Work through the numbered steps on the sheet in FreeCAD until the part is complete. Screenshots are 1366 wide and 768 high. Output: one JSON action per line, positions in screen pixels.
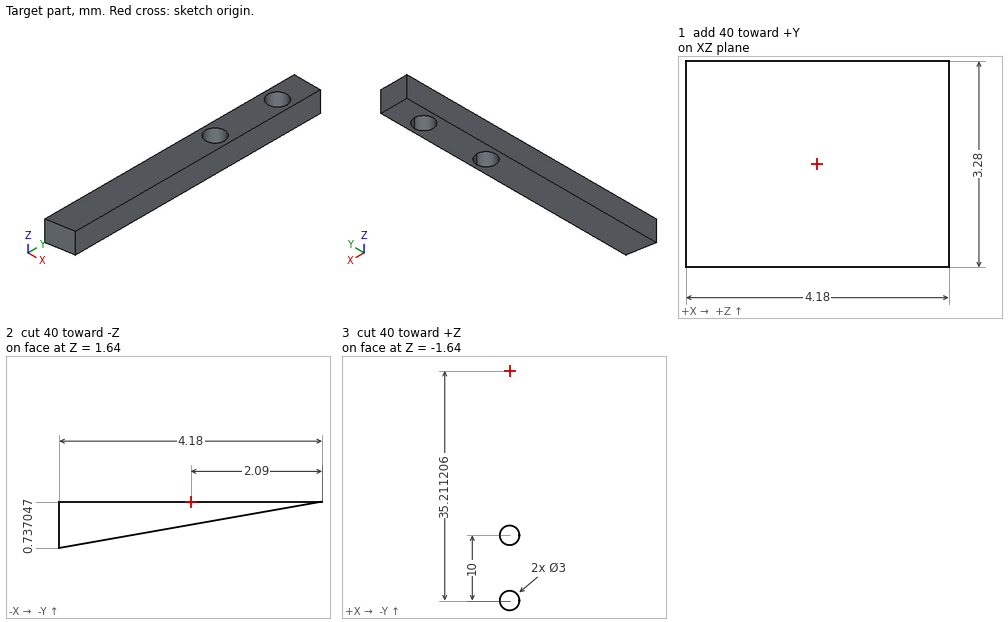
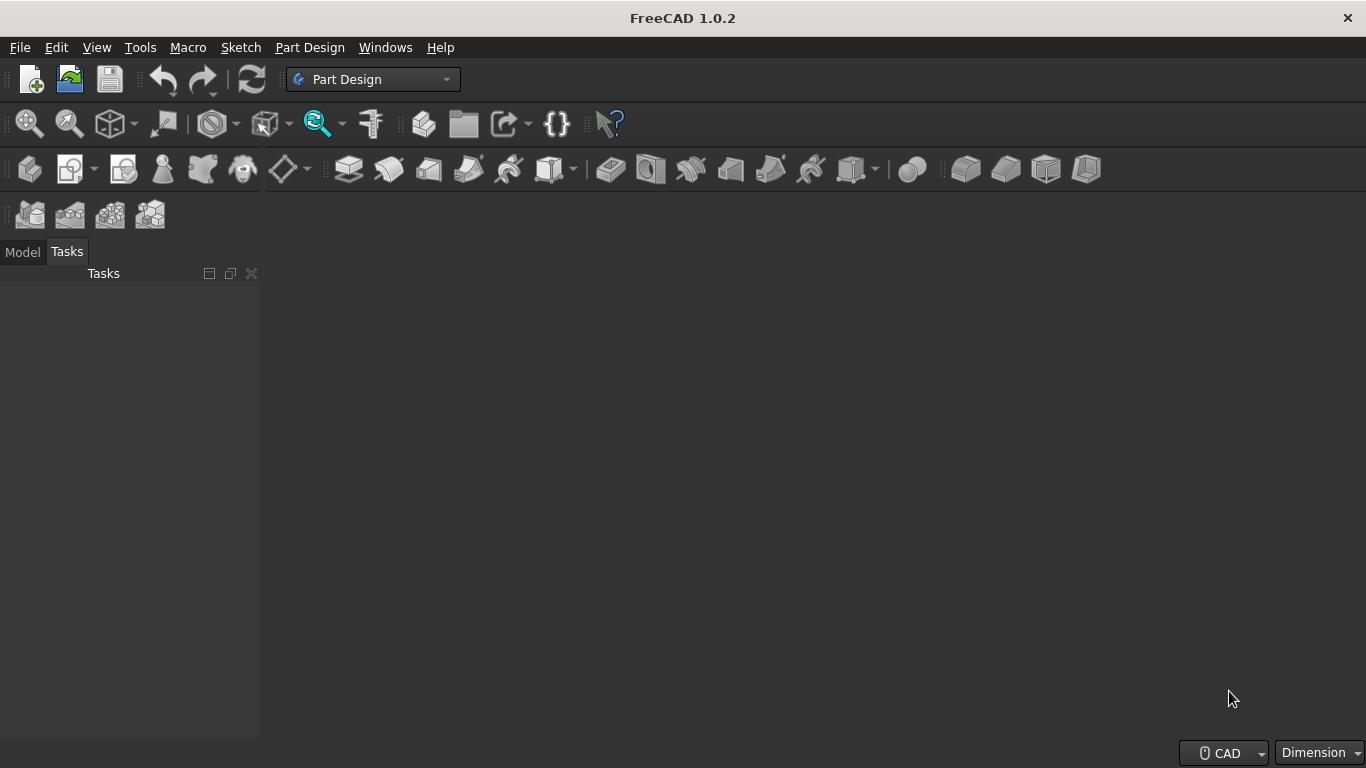
{"action": "left_click", "coordinate": [30, 80]}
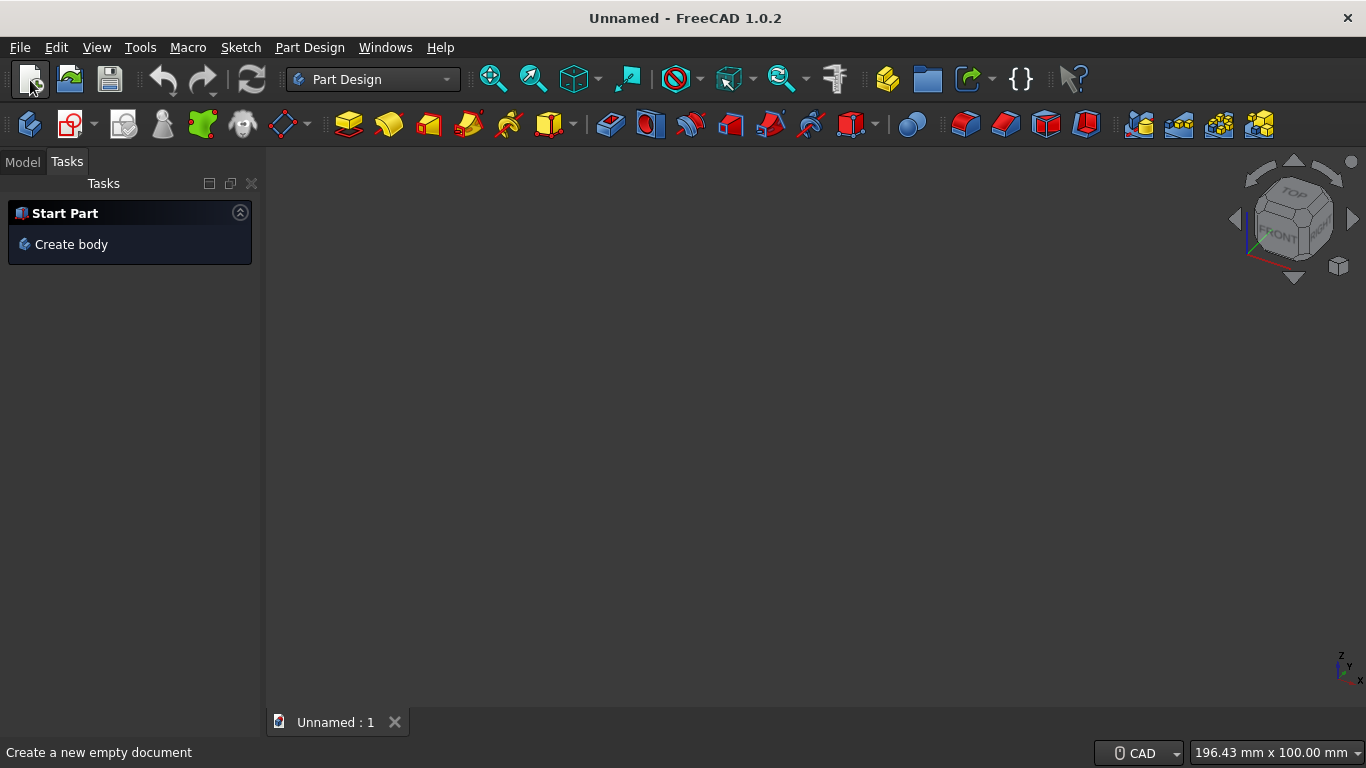
{"action": "left_click", "coordinate": [70, 124]}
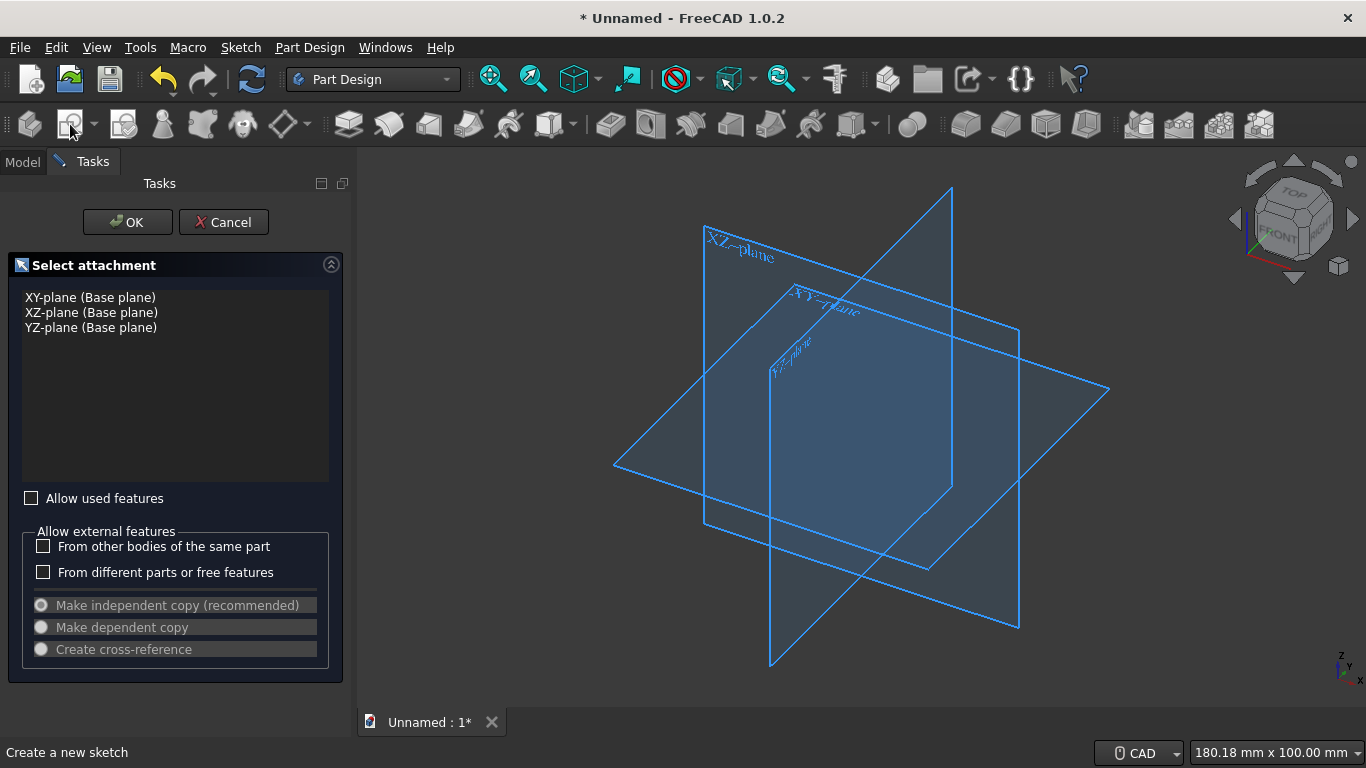
{"action": "left_click", "coordinate": [82, 312]}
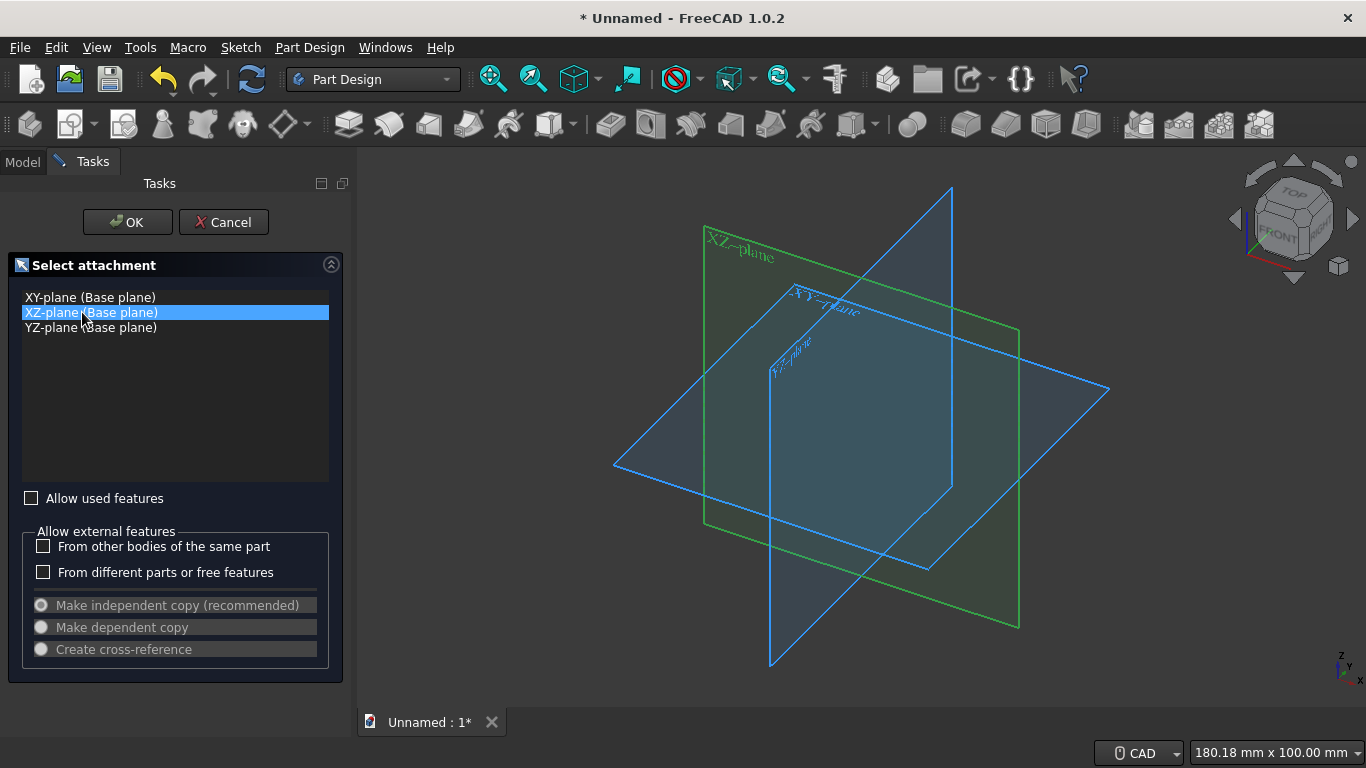
{"action": "left_click", "coordinate": [128, 222]}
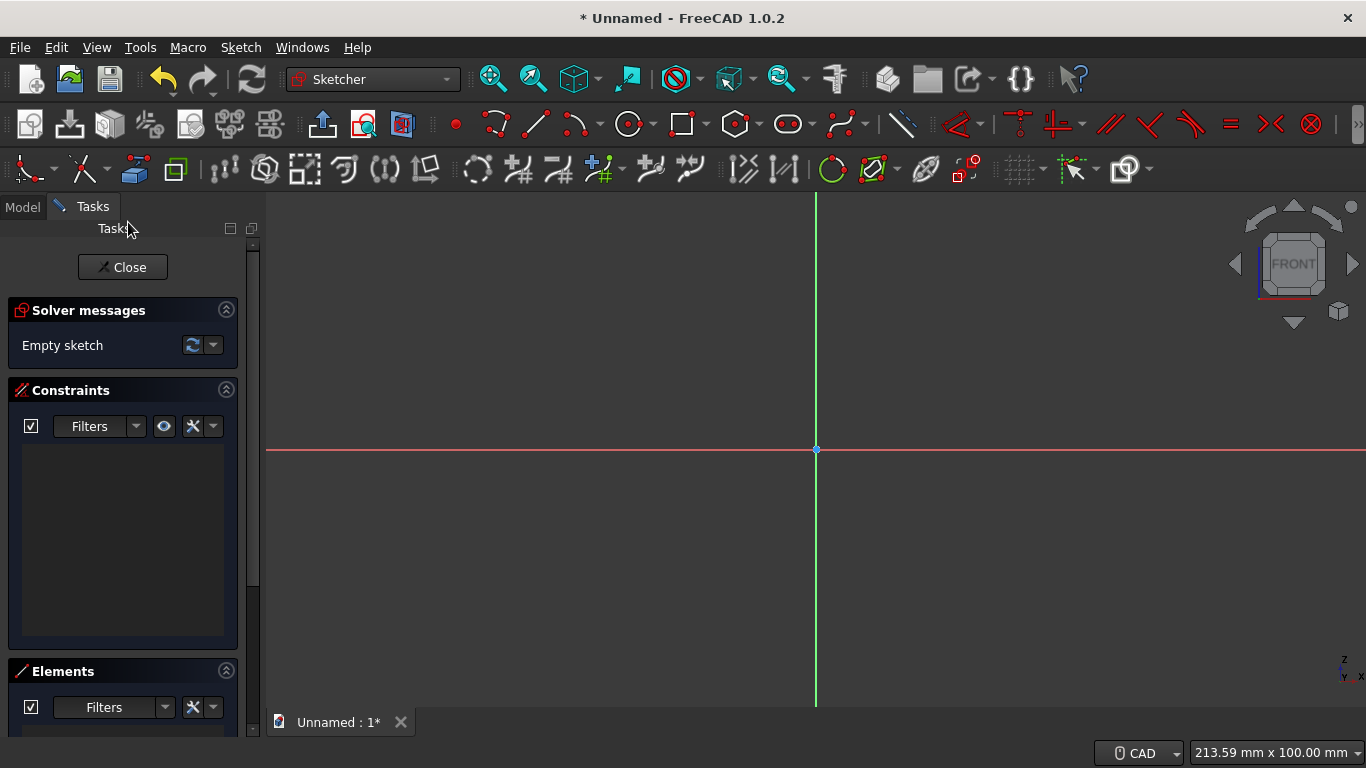
{"action": "scroll", "coordinate": [820, 450], "scroll_direction": "up", "scroll_amount": 15}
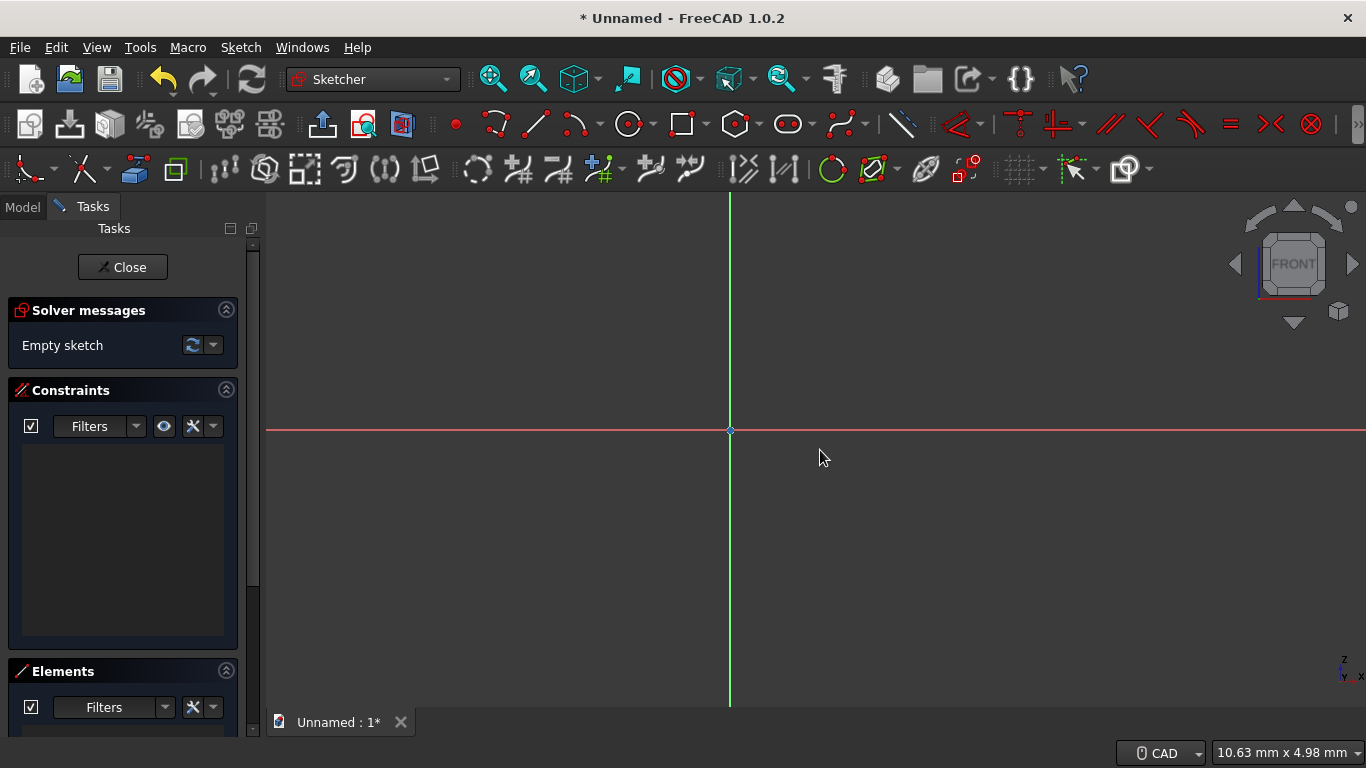
{"action": "key", "text": "g v"}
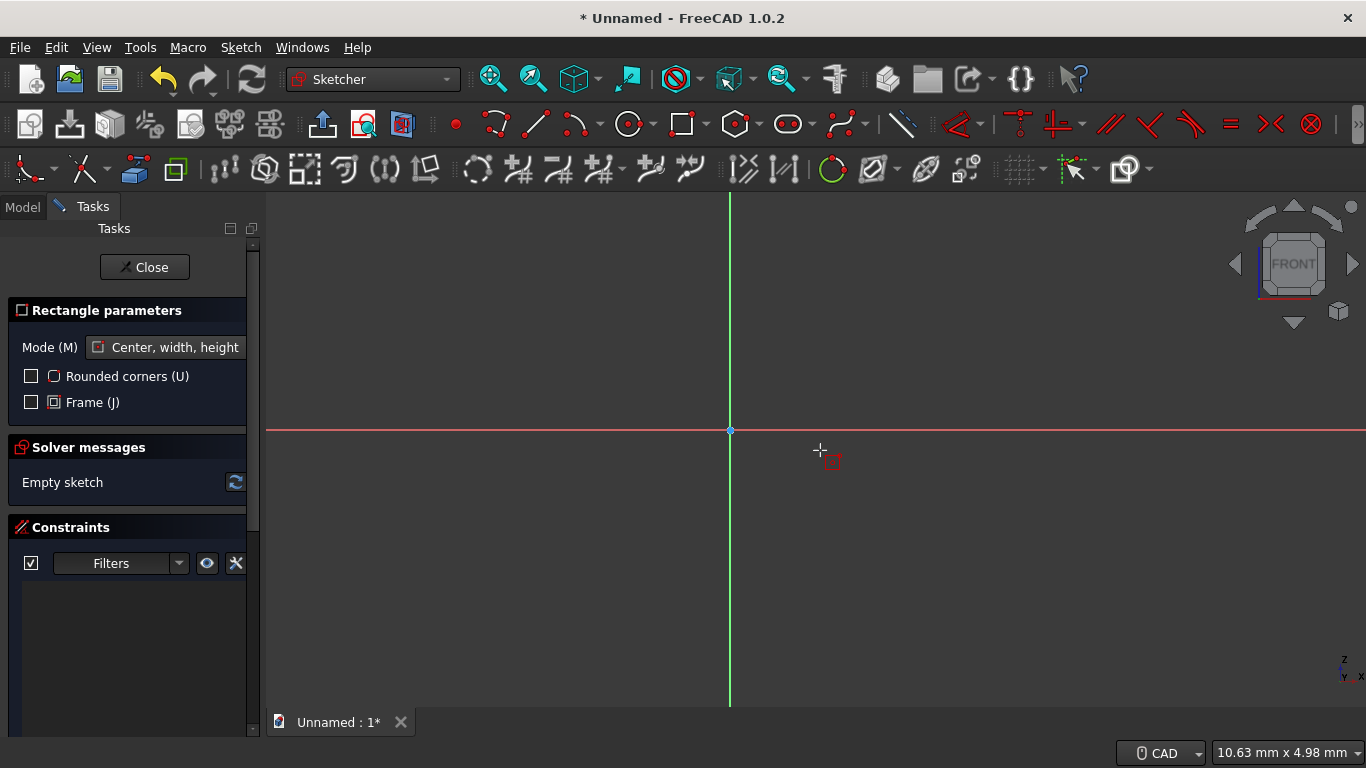
{"action": "left_click", "coordinate": [730, 430]}
{"action": "mouse_move", "coordinate": [946, 261]}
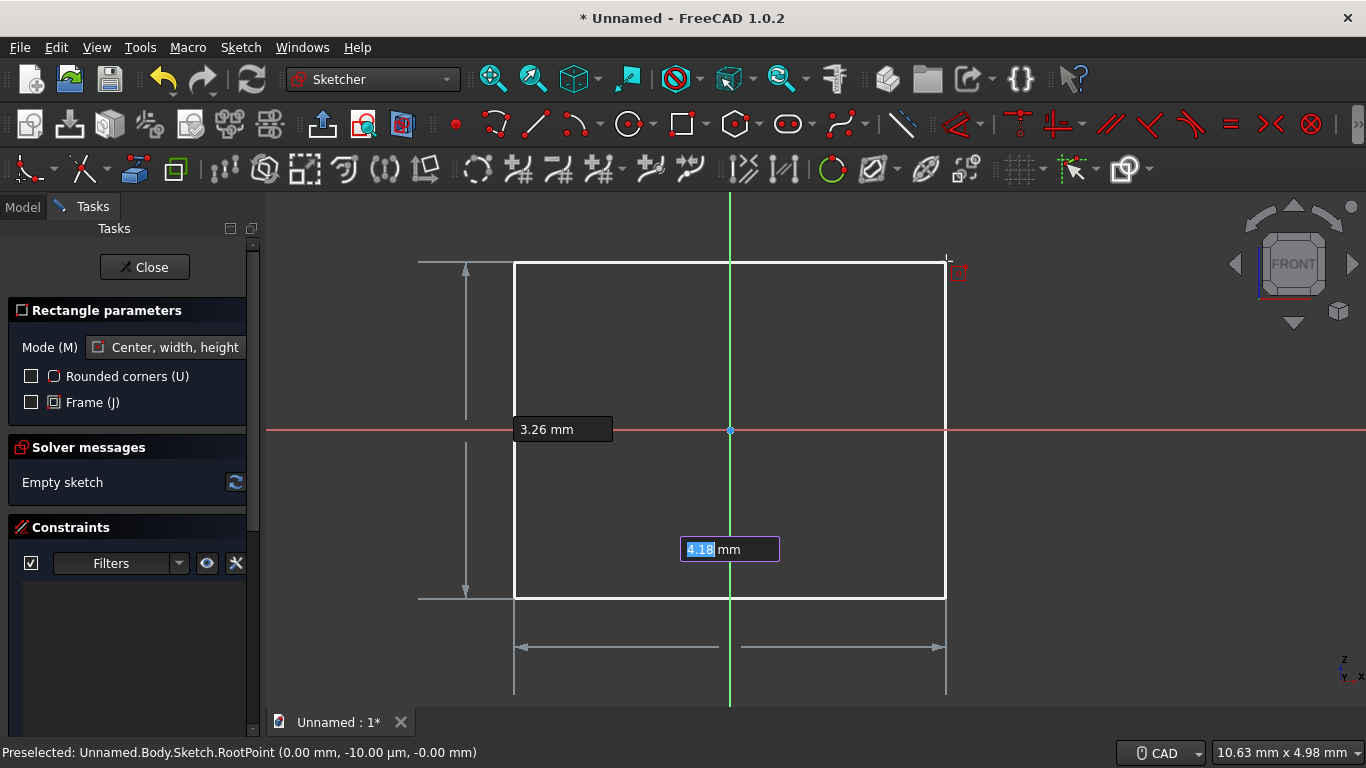
{"action": "type", "text": "4.18"}
{"action": "key", "text": "Tab"}
{"action": "type", "text": "3.28"}
{"action": "key", "text": "Return"}
{"action": "key", "text": "Escape"}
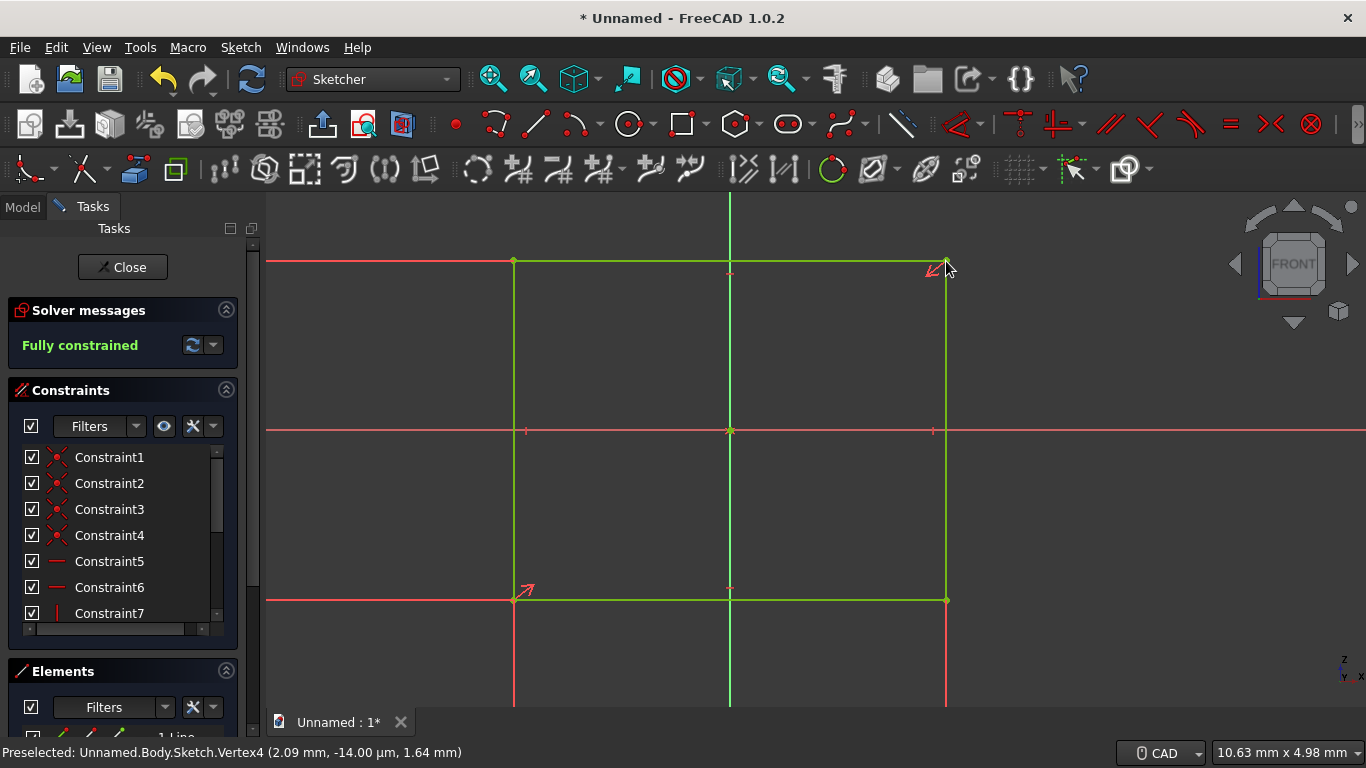
{"action": "left_click", "coordinate": [123, 267]}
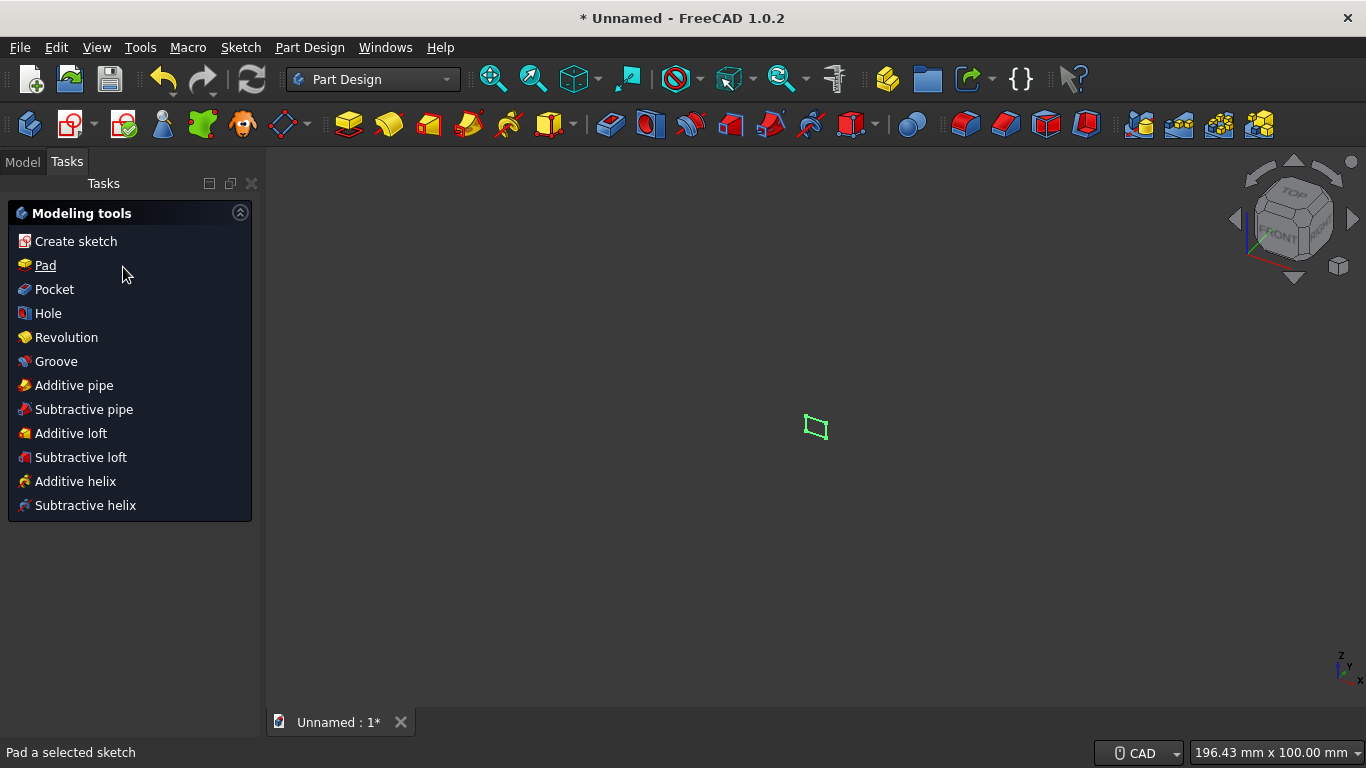
{"action": "left_click", "coordinate": [350, 124]}